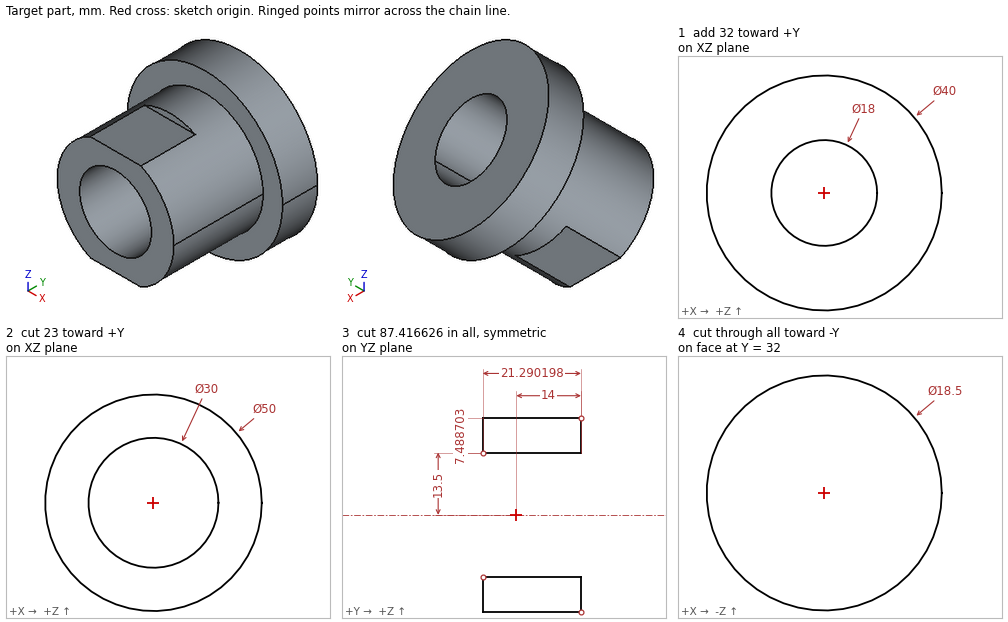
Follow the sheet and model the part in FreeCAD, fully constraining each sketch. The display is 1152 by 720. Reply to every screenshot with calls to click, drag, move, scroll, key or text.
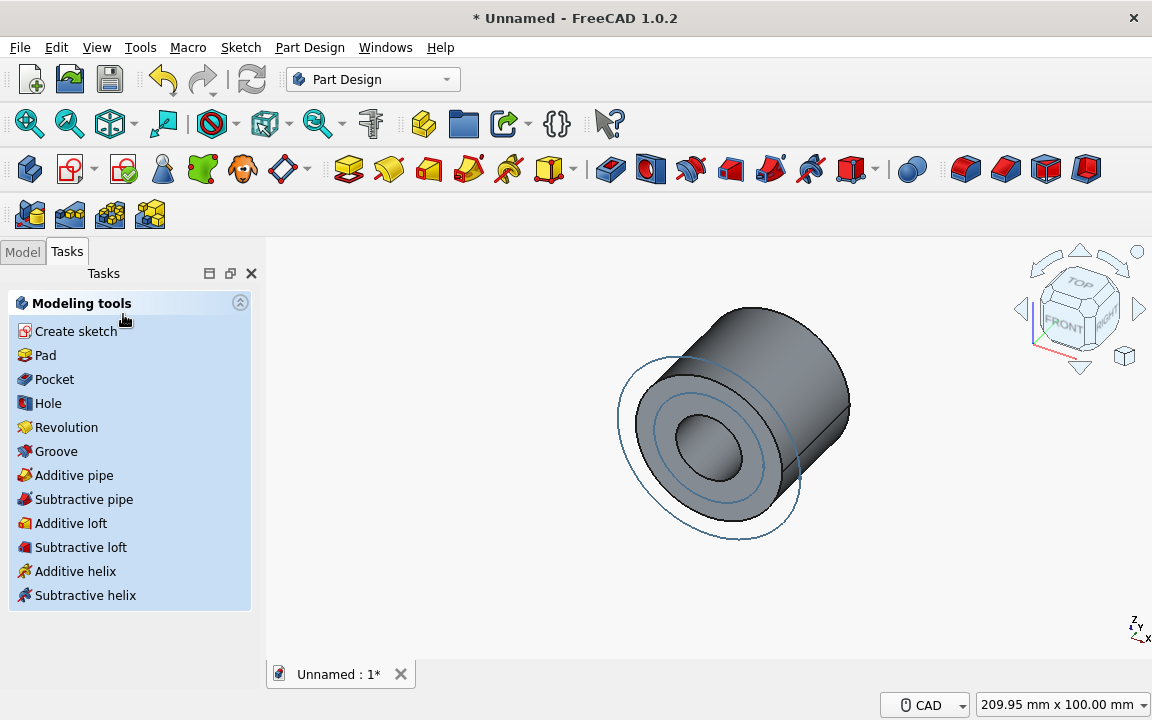
click(612, 170)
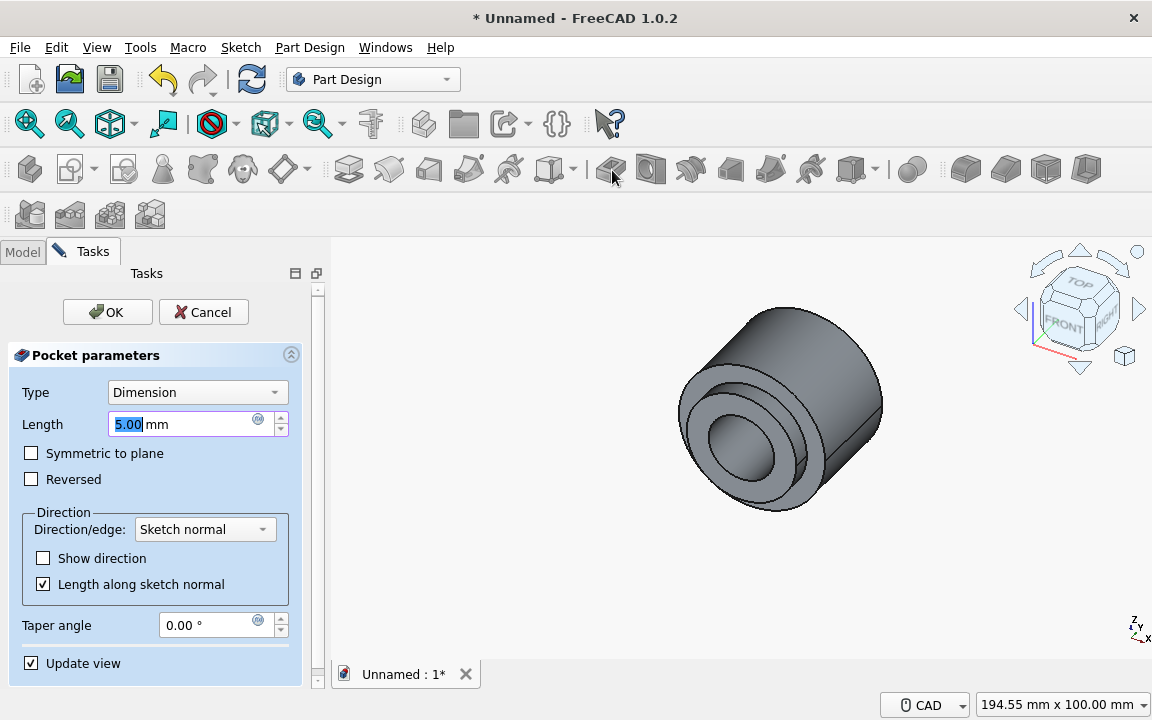
text(23)
key(Tab)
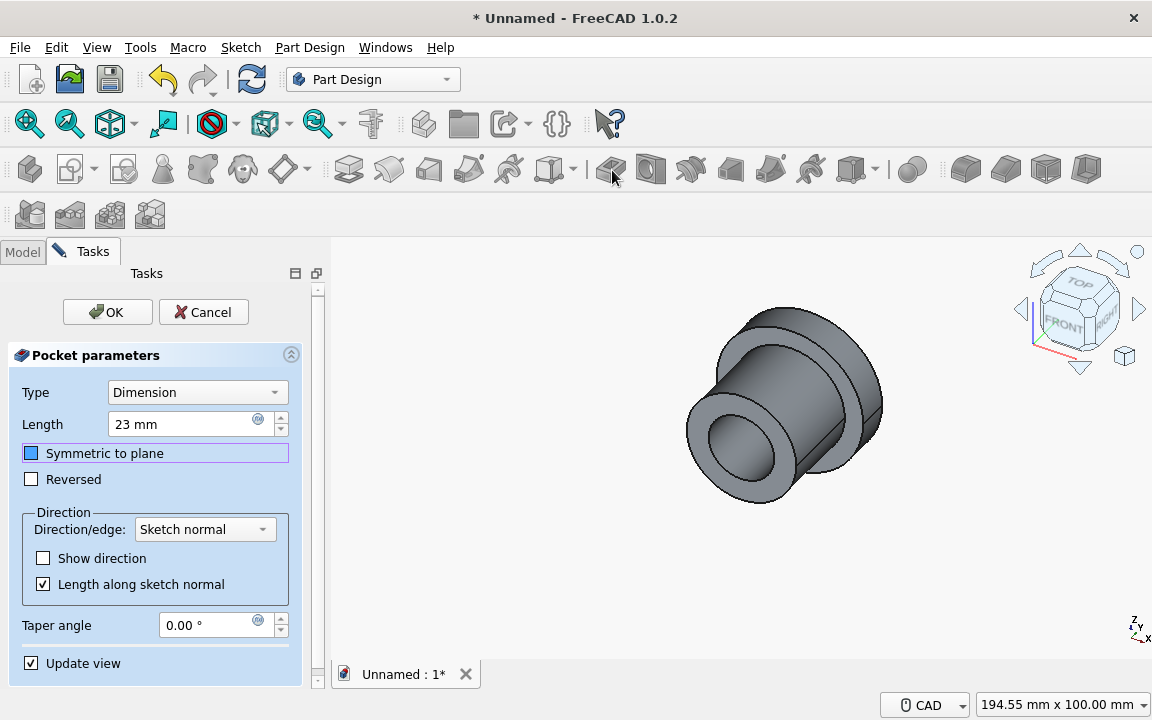
click(108, 312)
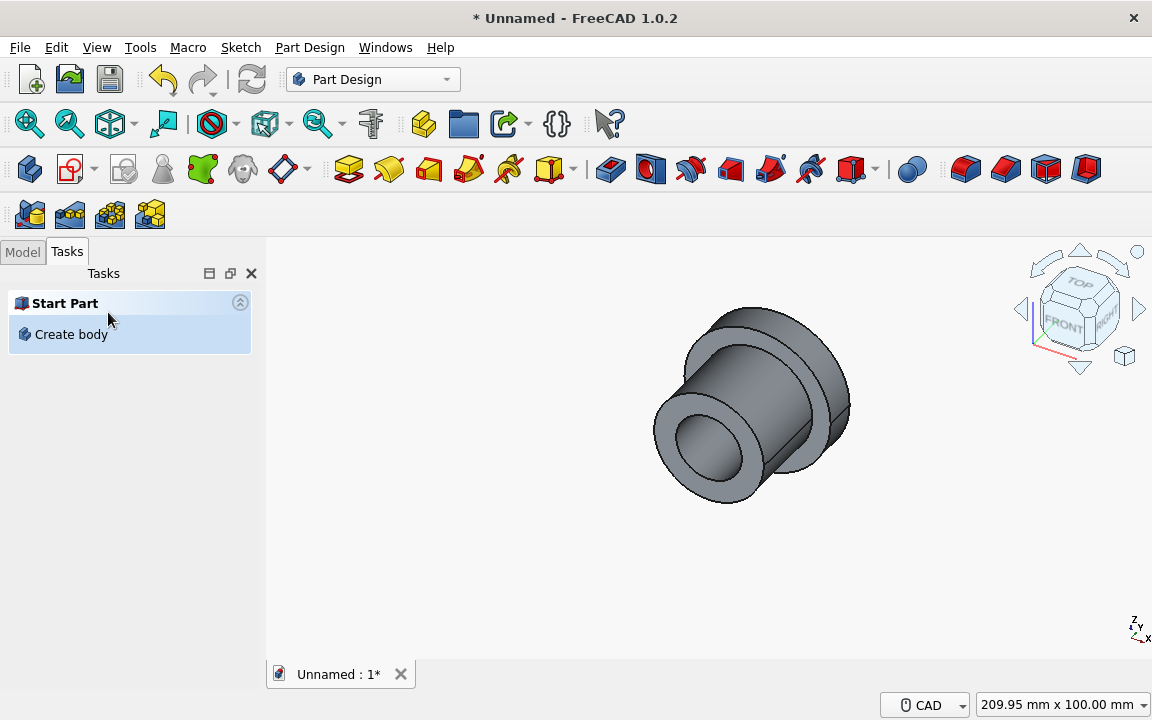
click(70, 170)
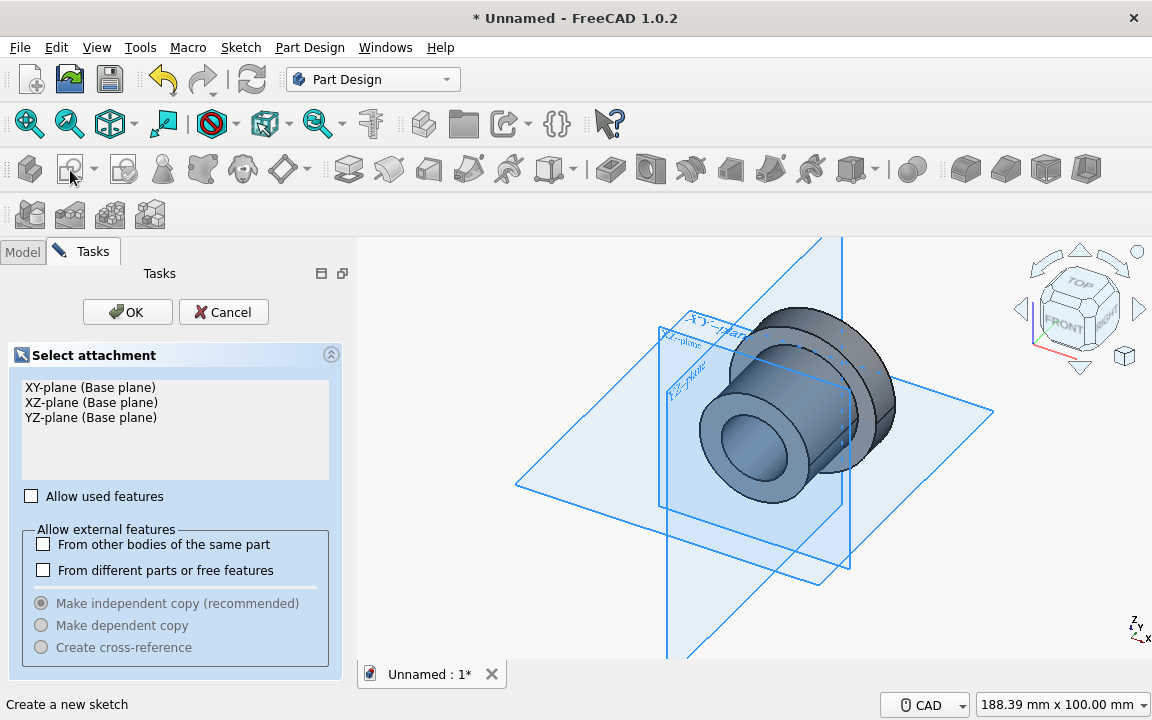
click(82, 418)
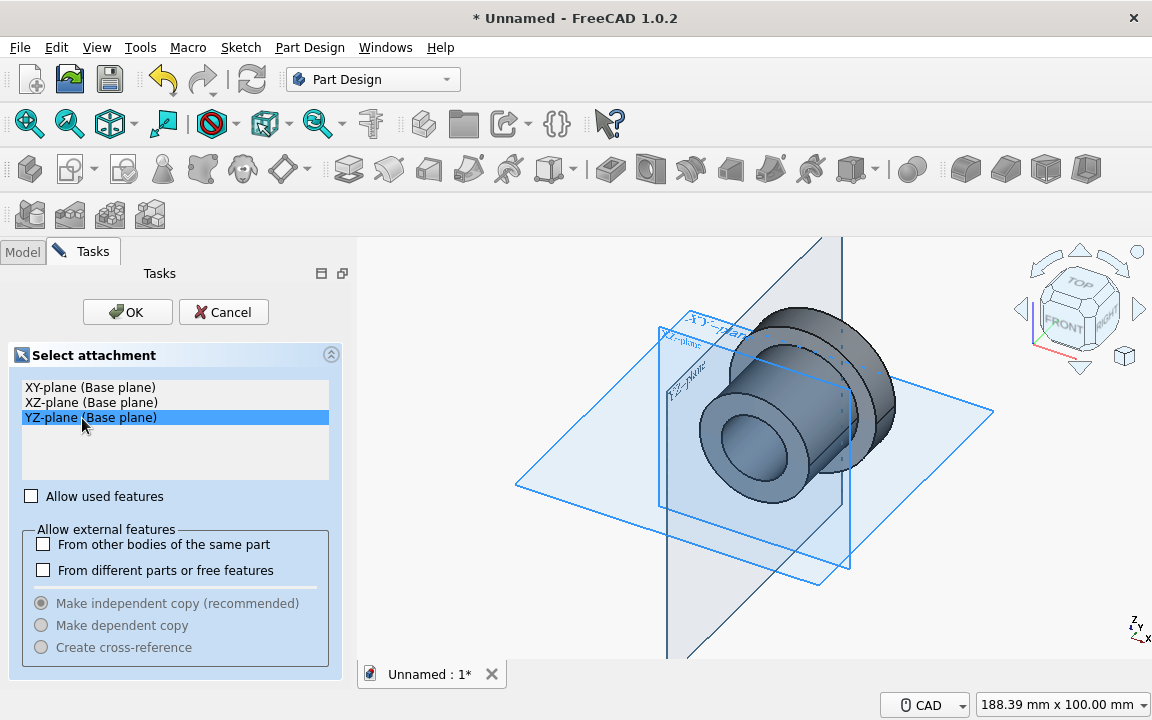
click(128, 312)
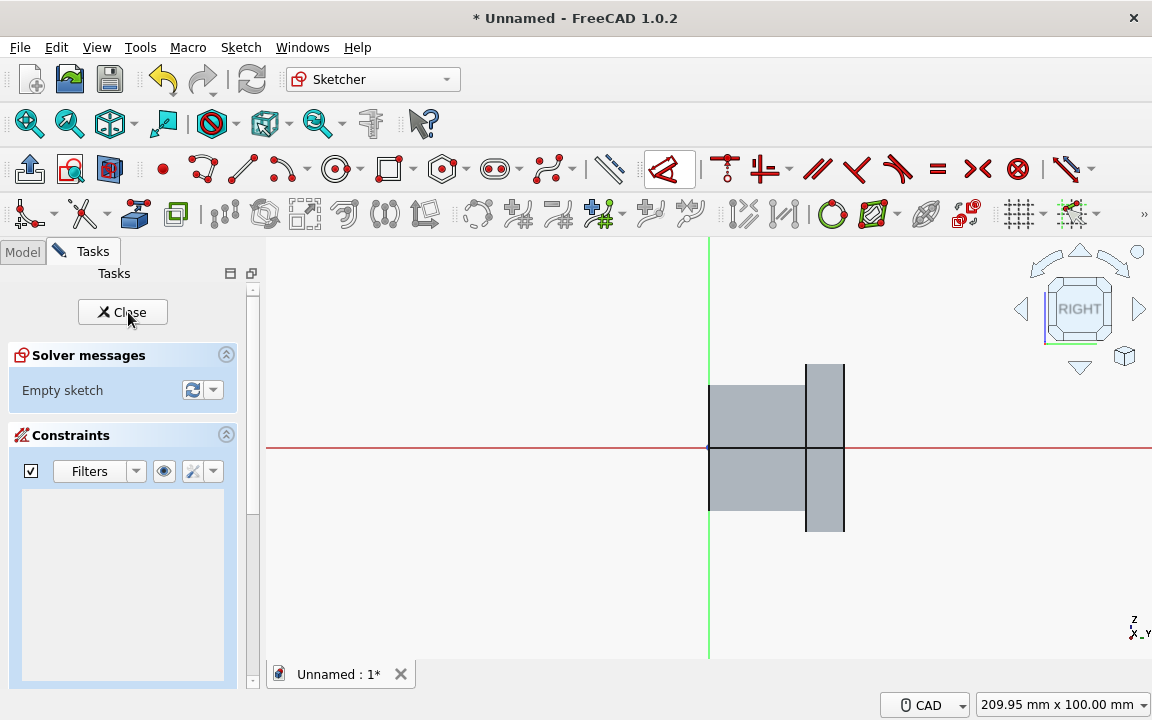
click(110, 170)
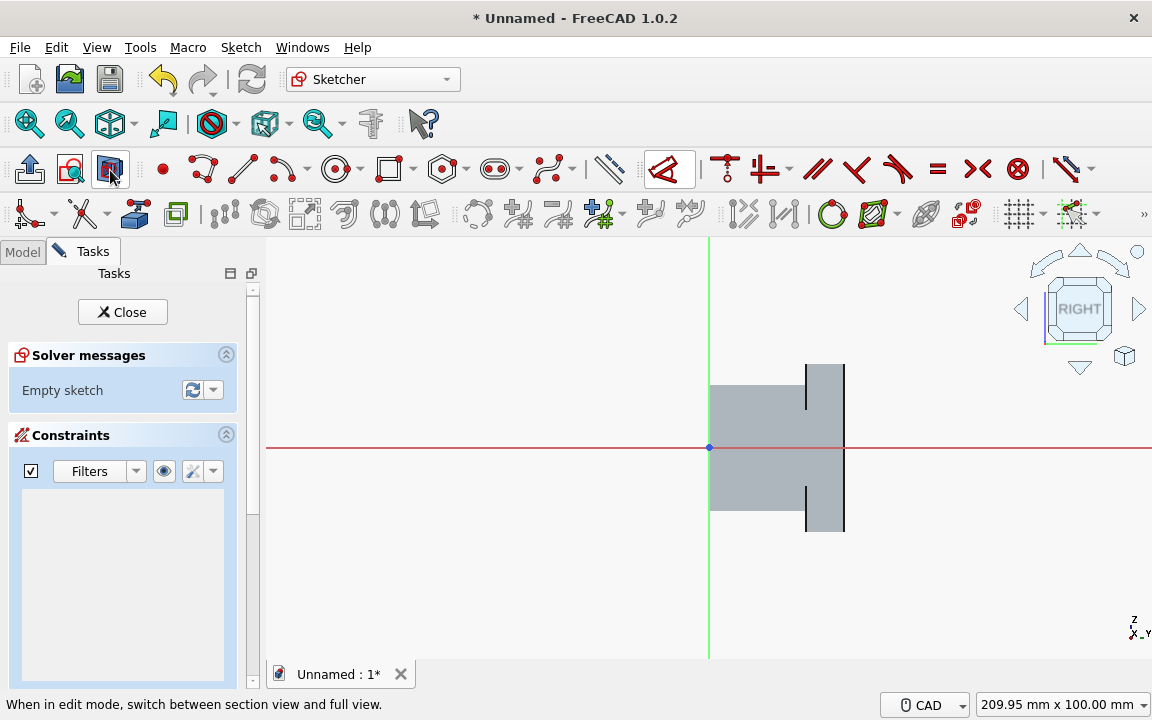
scroll(891, 448, up, 2)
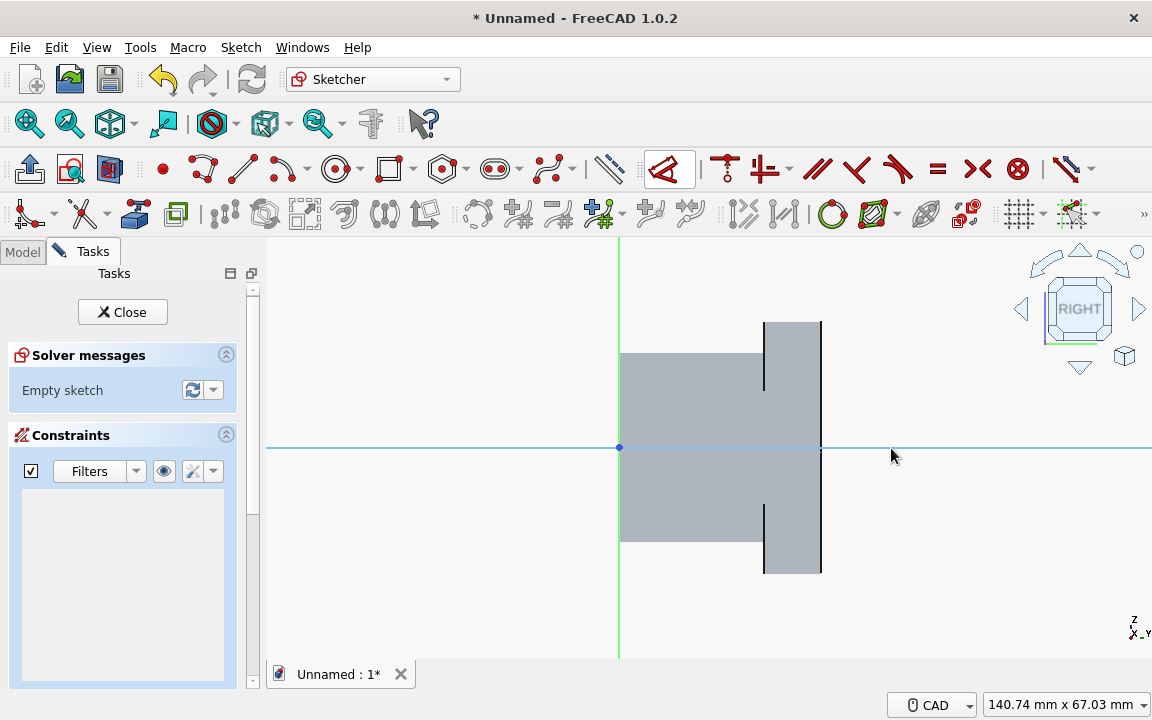
key(g)
key(r)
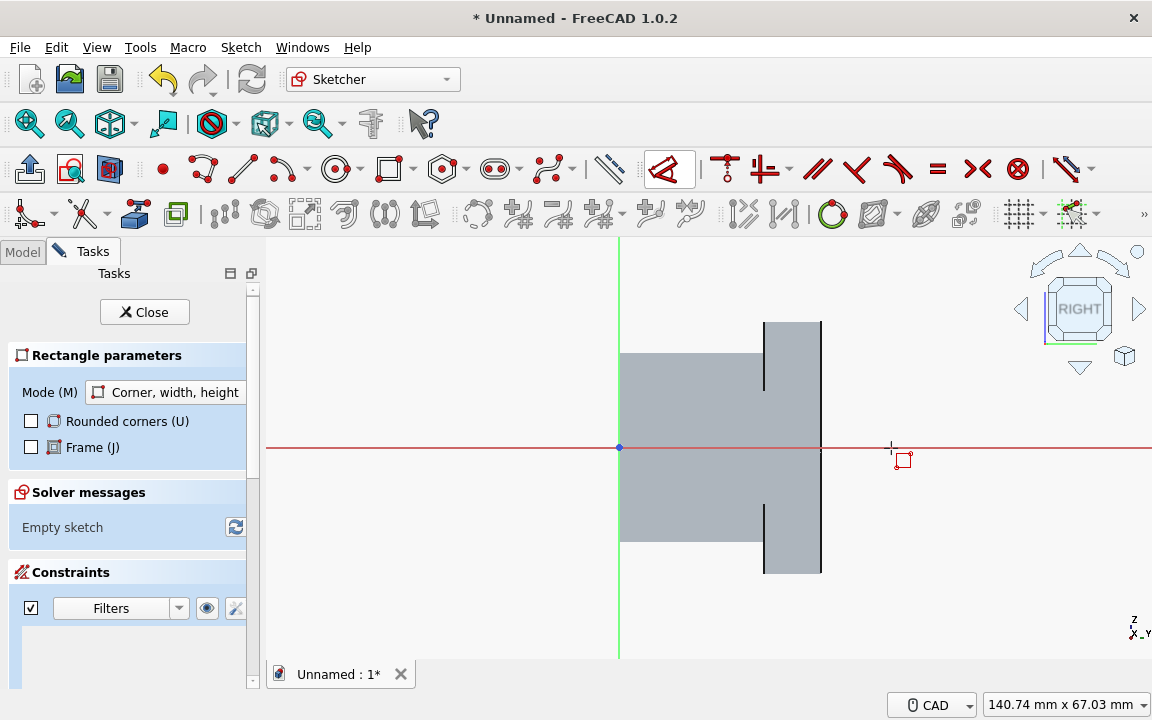
click(573, 316)
click(707, 363)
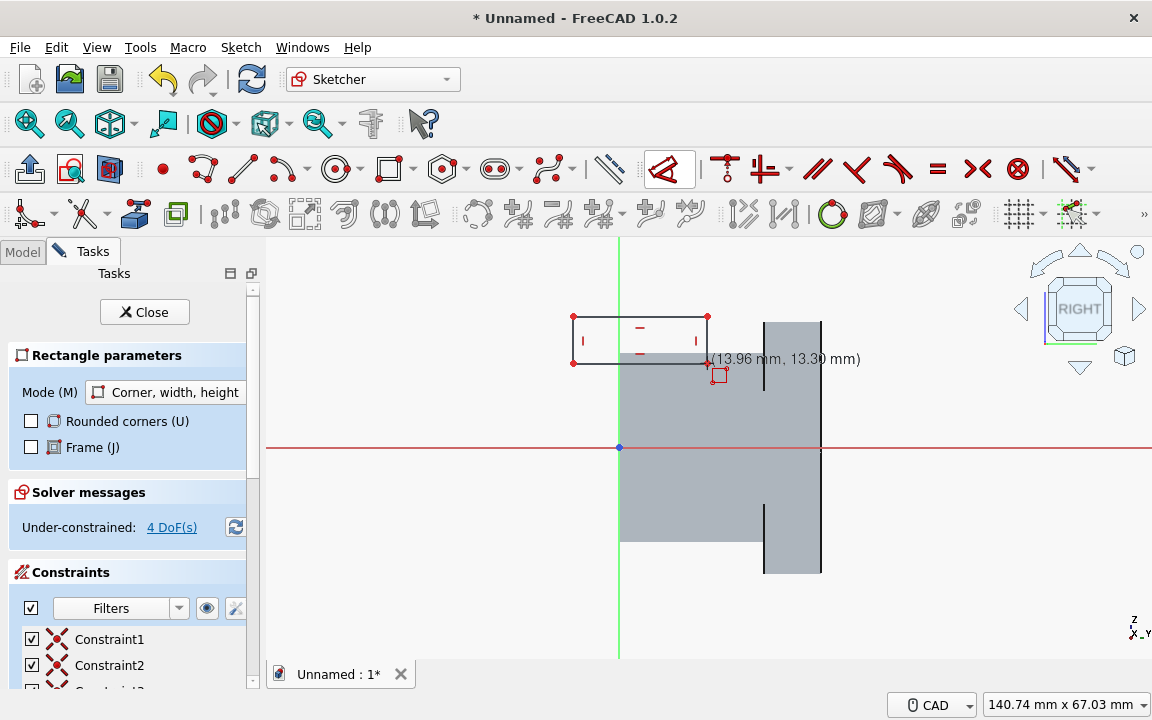
click(573, 533)
click(707, 580)
key(Escape)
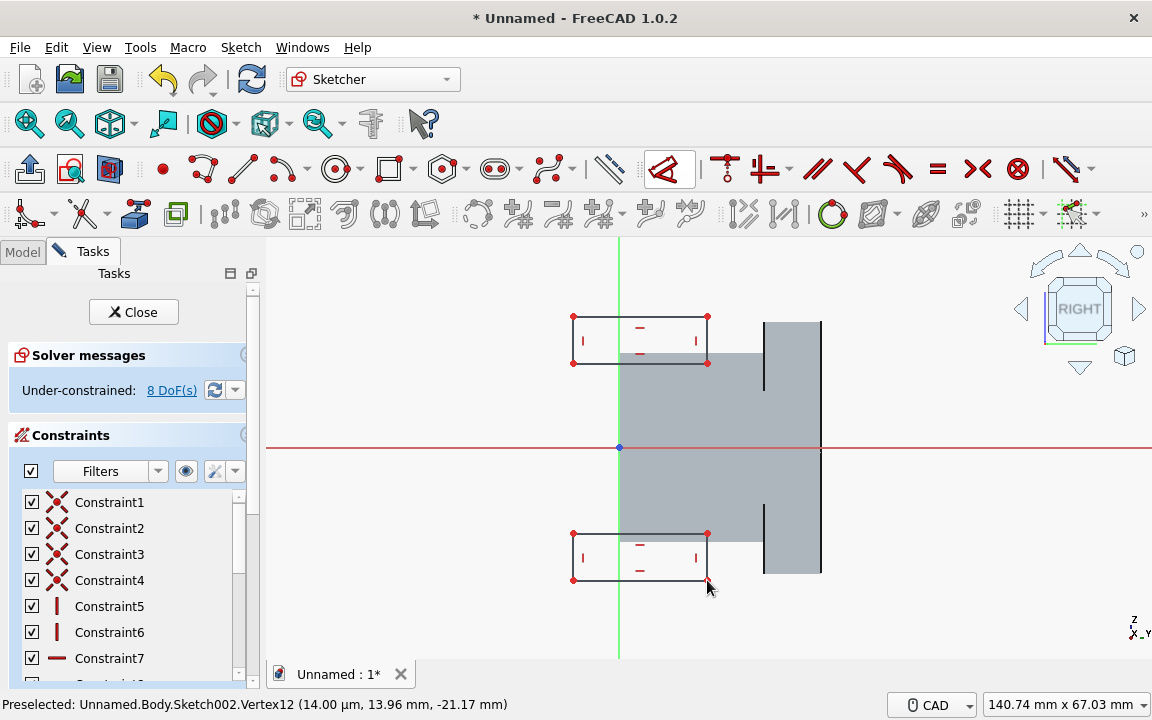
click(573, 364)